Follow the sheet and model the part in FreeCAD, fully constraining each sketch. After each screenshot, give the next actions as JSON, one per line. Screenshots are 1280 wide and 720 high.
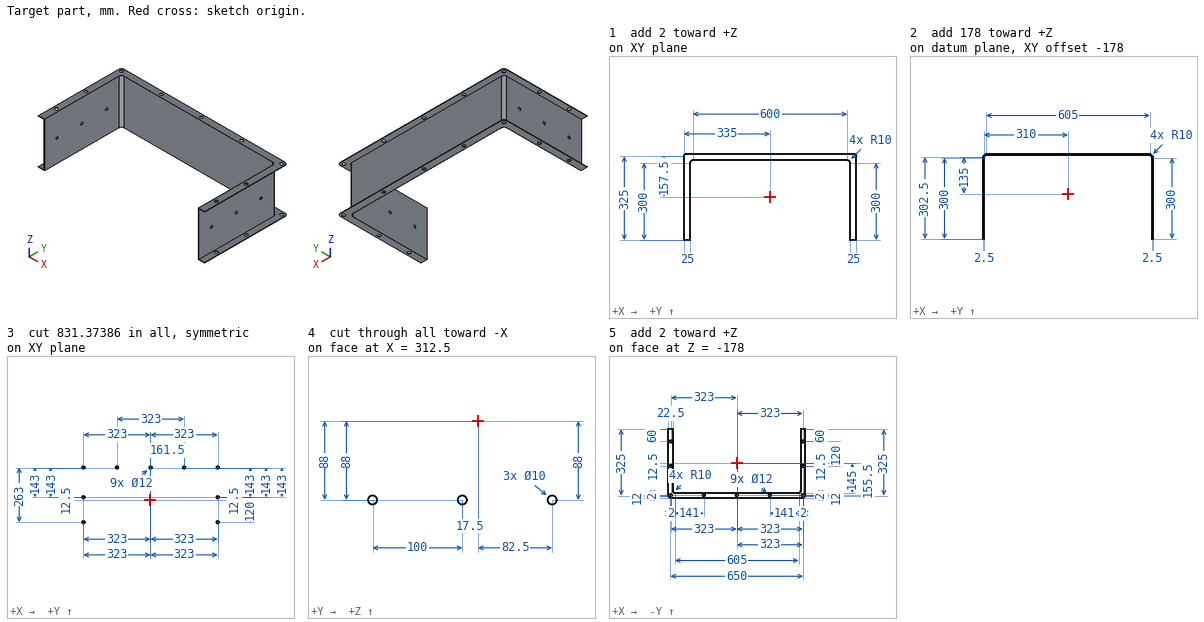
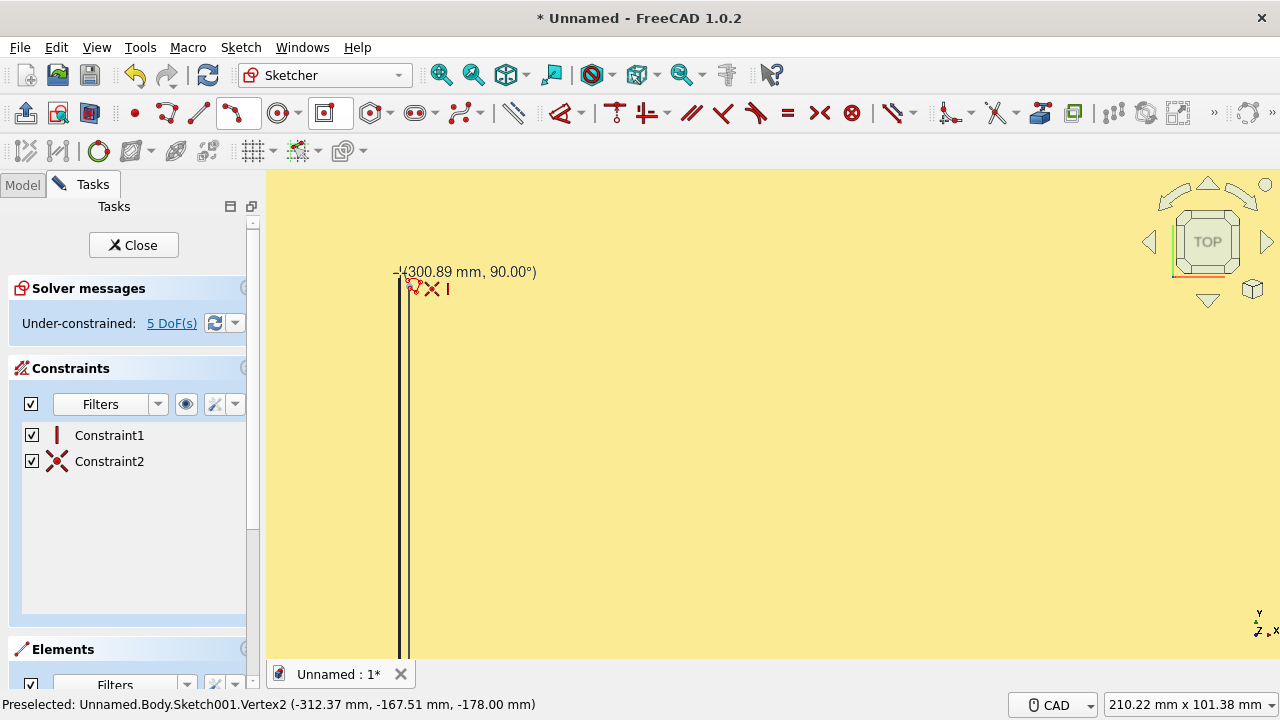
{"action": "left_click", "coordinate": [399, 270]}
{"action": "right_click", "coordinate": [399, 270]}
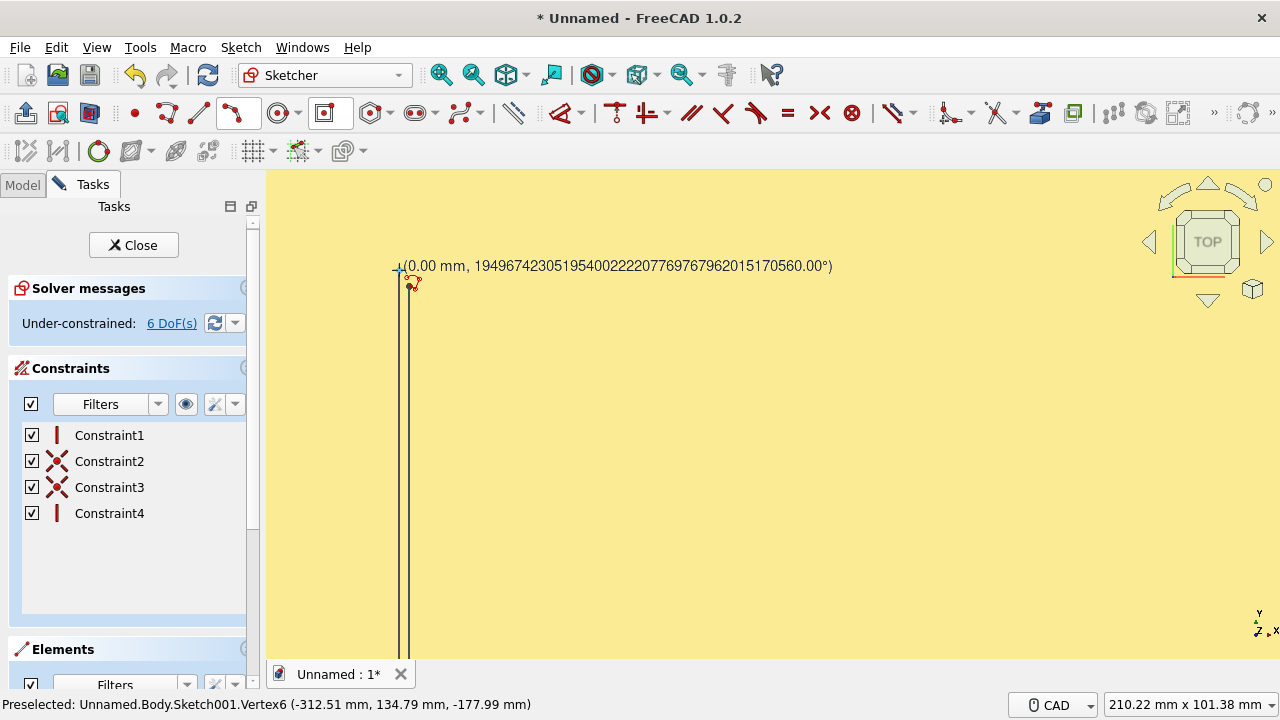
{"action": "left_click", "coordinate": [200, 114]}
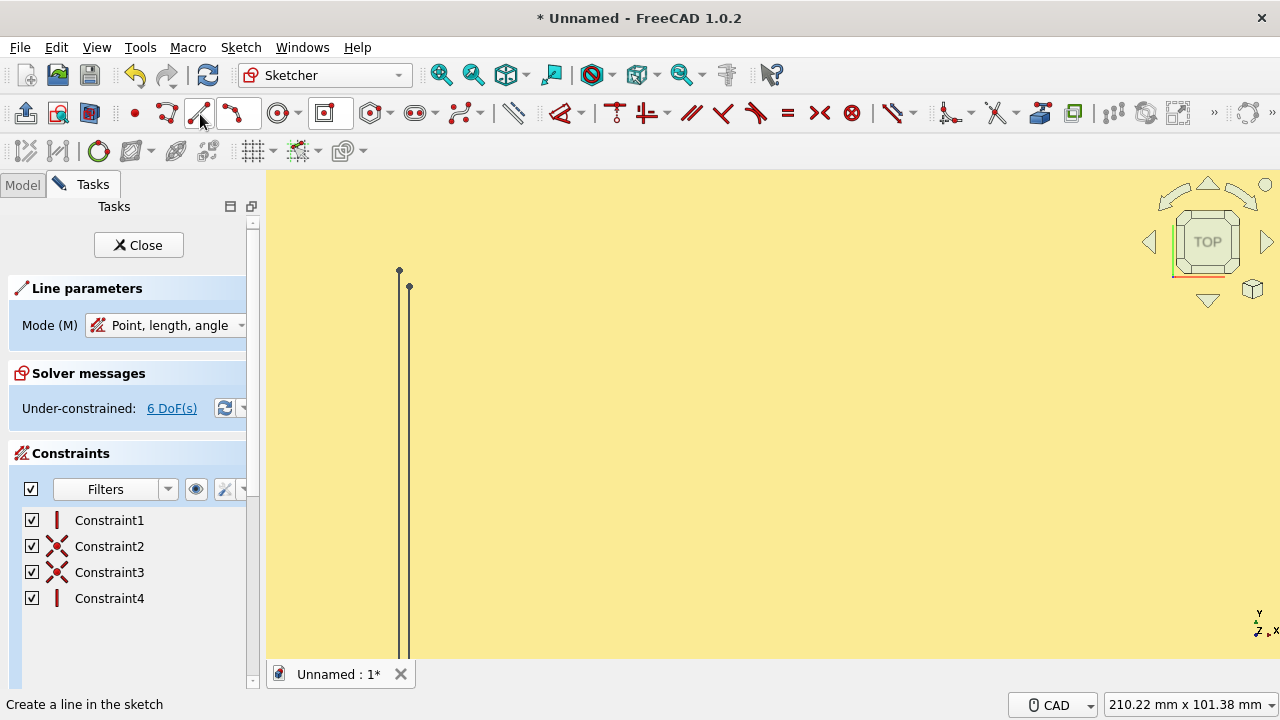
{"action": "scroll", "coordinate": [400, 273], "scroll_direction": "down", "scroll_amount": 8}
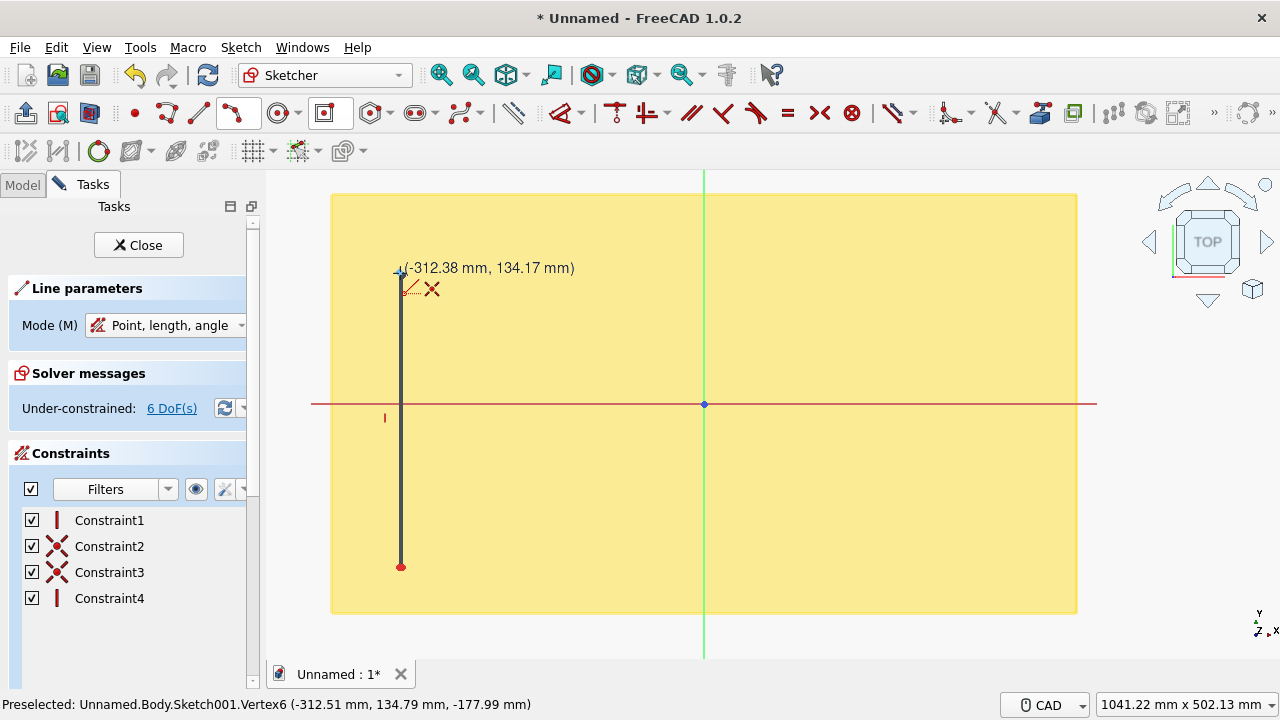
{"action": "left_click", "coordinate": [410, 263]}
{"action": "left_click", "coordinate": [999, 263]}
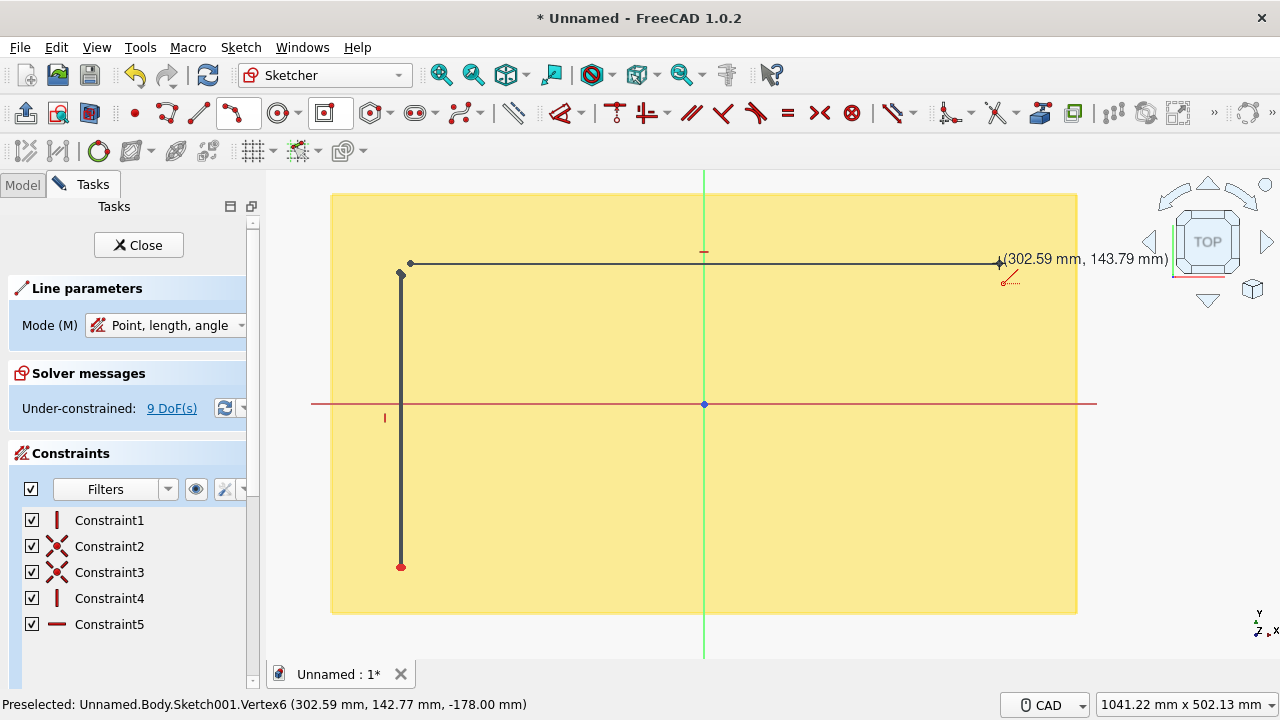
{"action": "left_click", "coordinate": [168, 114]}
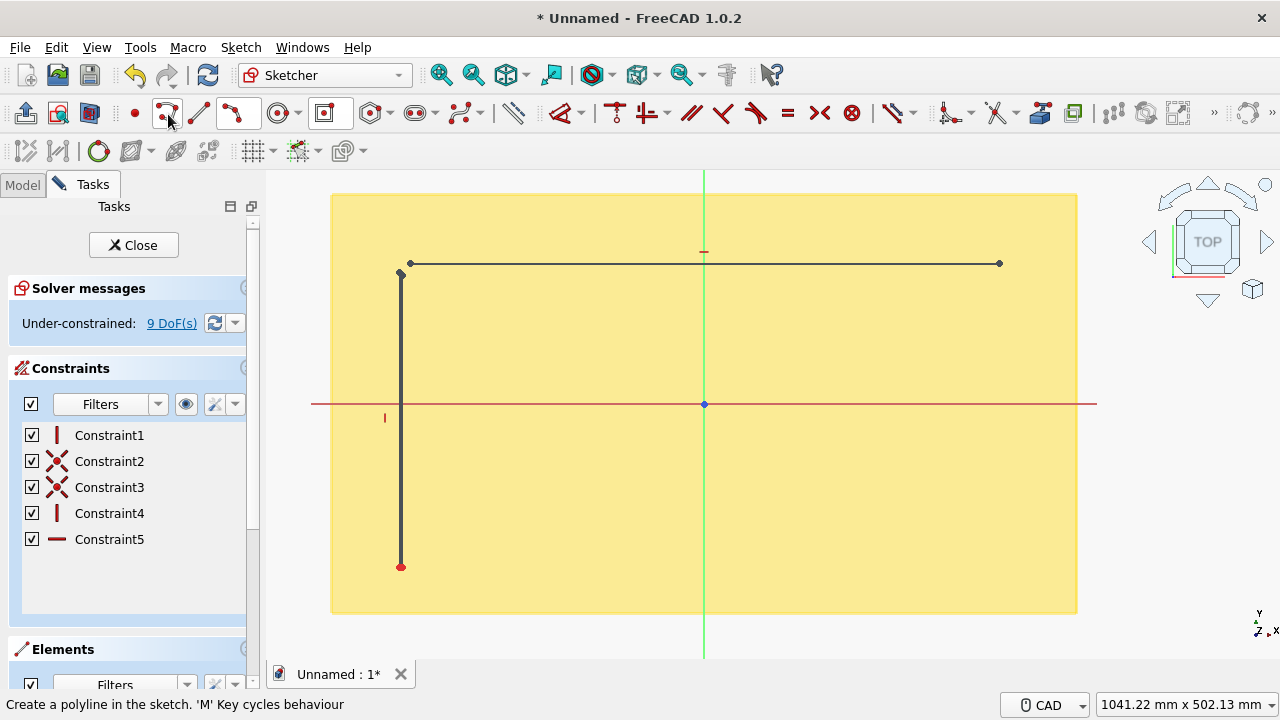
{"action": "left_click", "coordinate": [1009, 273]}
{"action": "left_click", "coordinate": [1009, 567]}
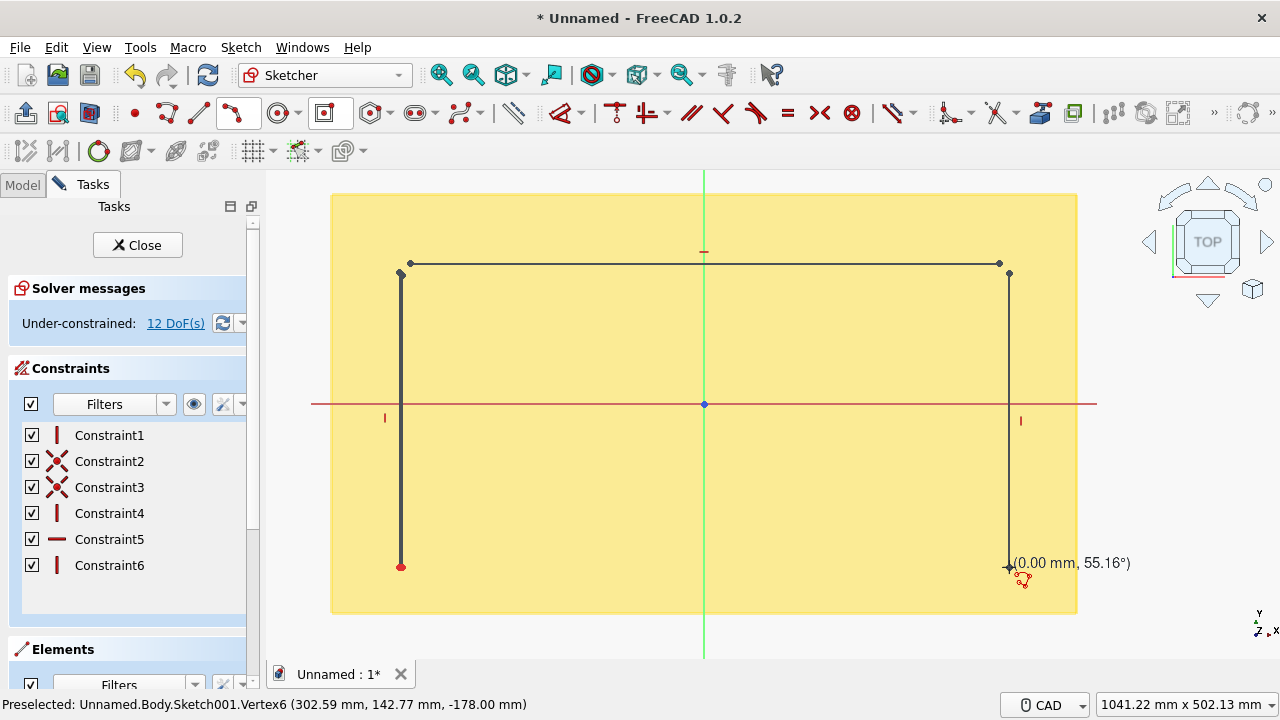
{"action": "scroll", "coordinate": [1006, 567], "scroll_direction": "up", "scroll_amount": 10}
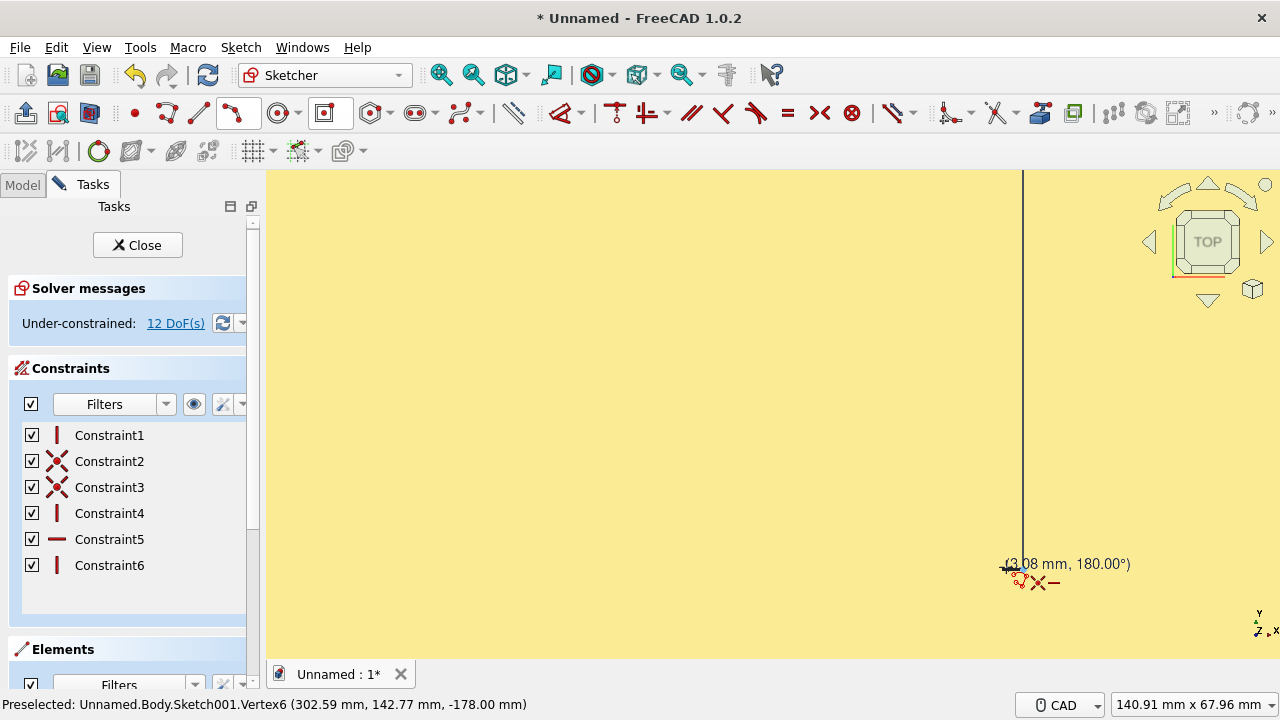
{"action": "left_click", "coordinate": [1003, 562]}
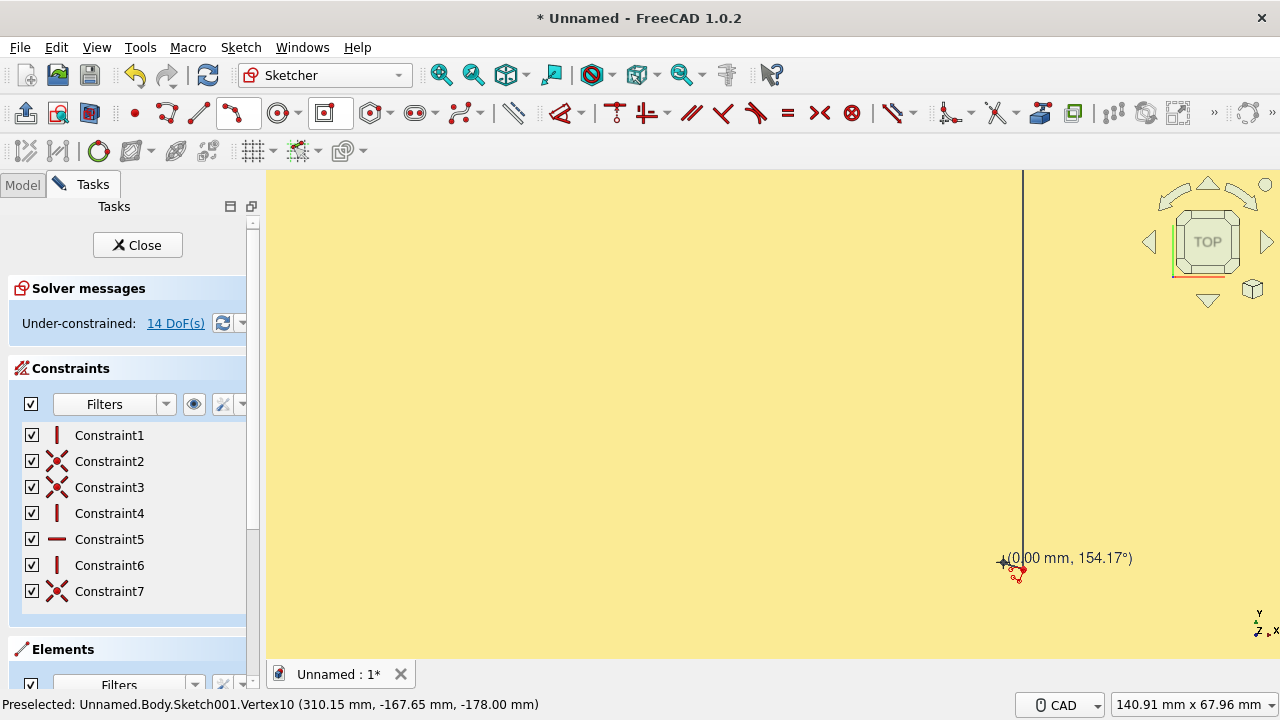
{"action": "scroll", "coordinate": [1007, 567], "scroll_direction": "down", "scroll_amount": 10}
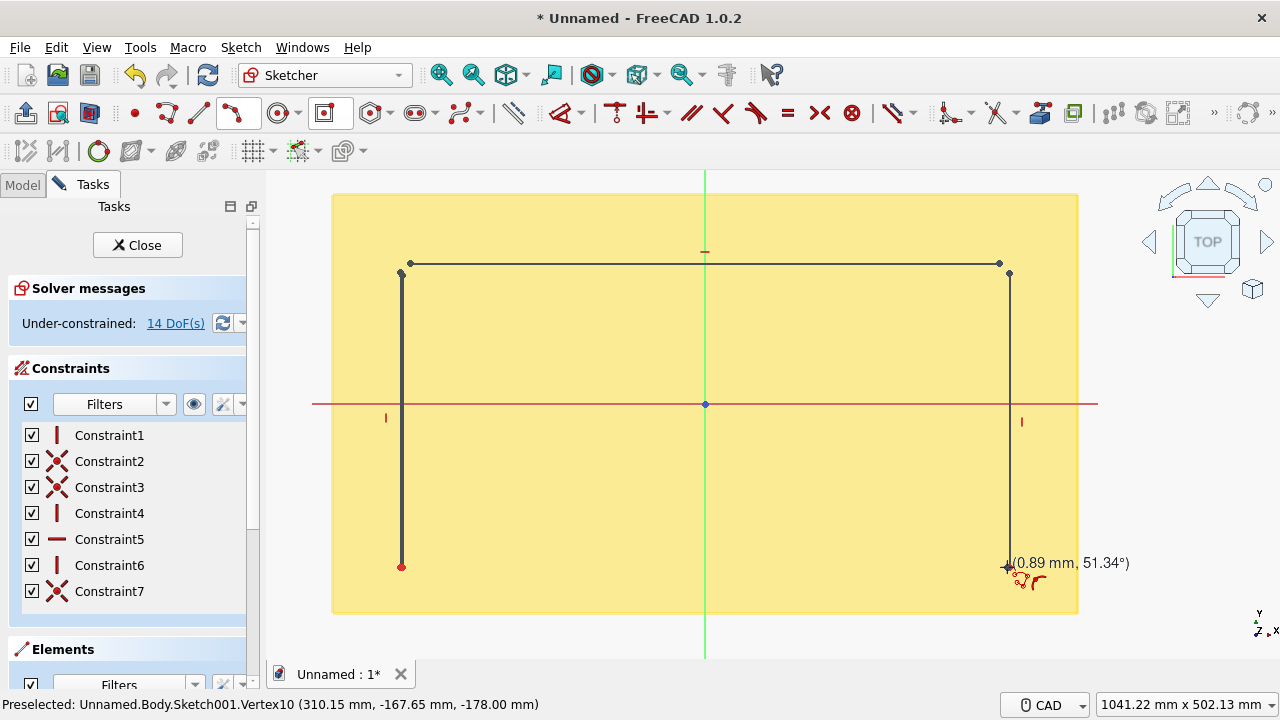
{"action": "scroll", "coordinate": [1007, 275], "scroll_direction": "up", "scroll_amount": 10}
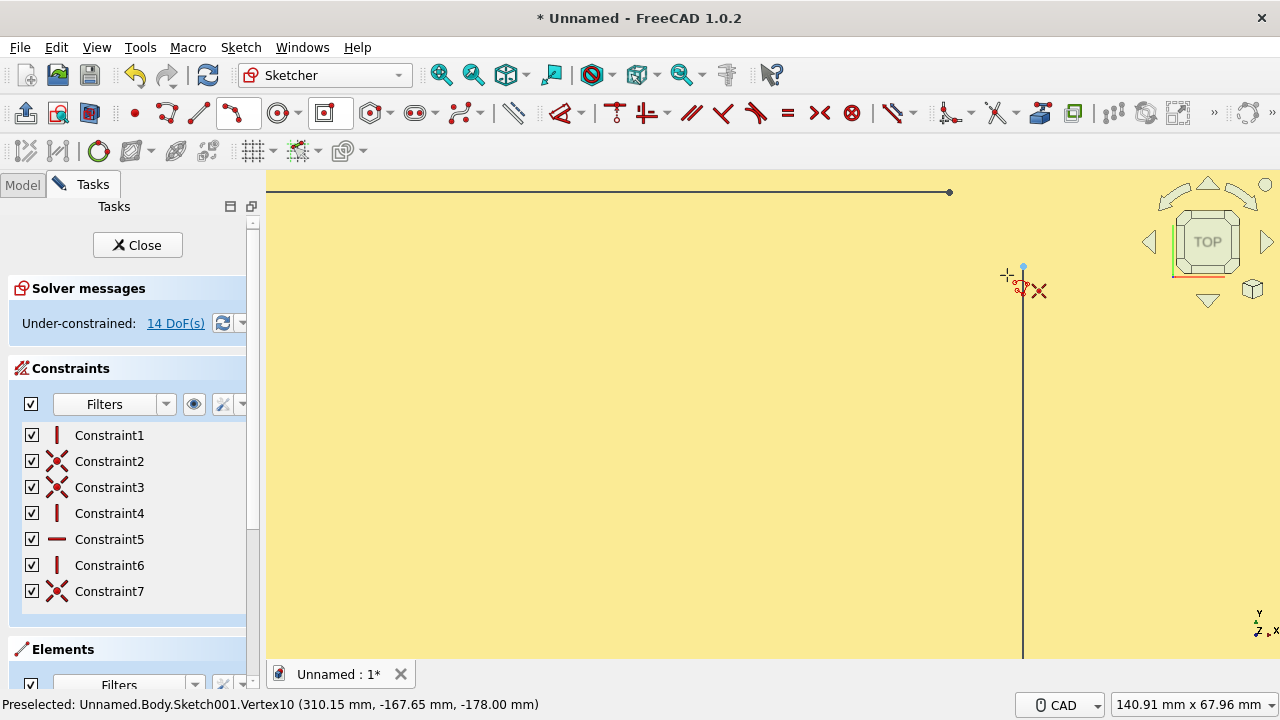
{"action": "left_click", "coordinate": [1003, 274]}
{"action": "right_click", "coordinate": [1003, 274]}